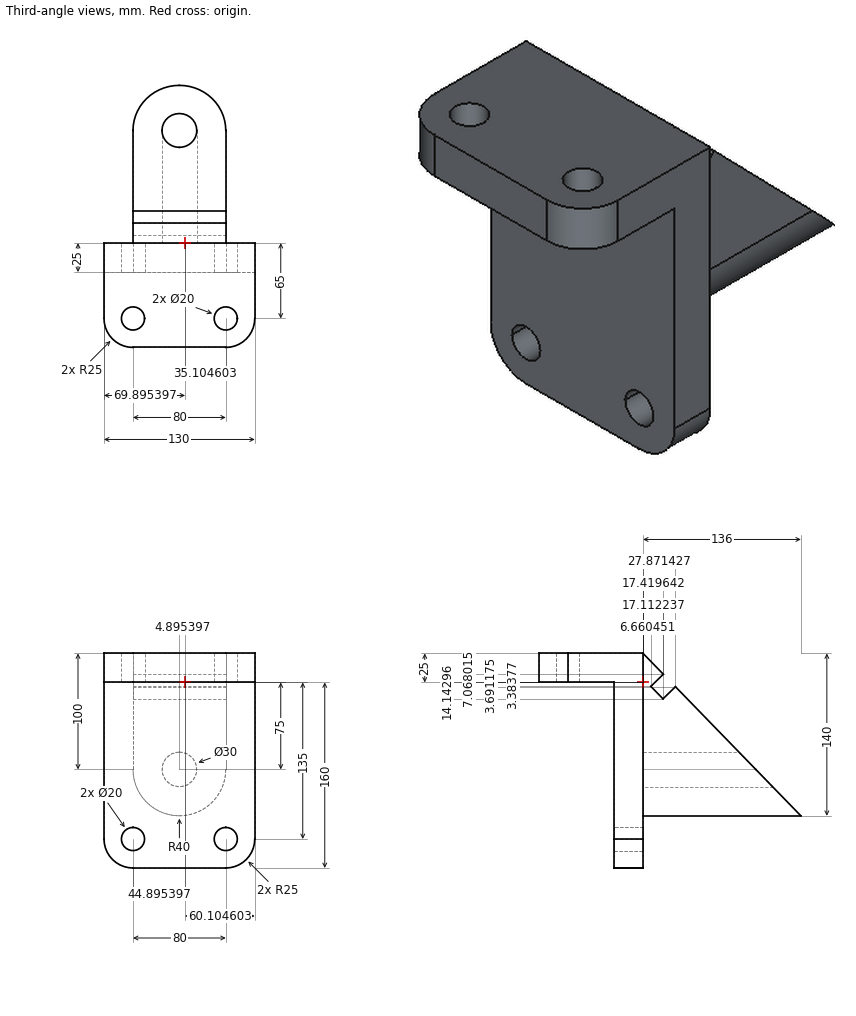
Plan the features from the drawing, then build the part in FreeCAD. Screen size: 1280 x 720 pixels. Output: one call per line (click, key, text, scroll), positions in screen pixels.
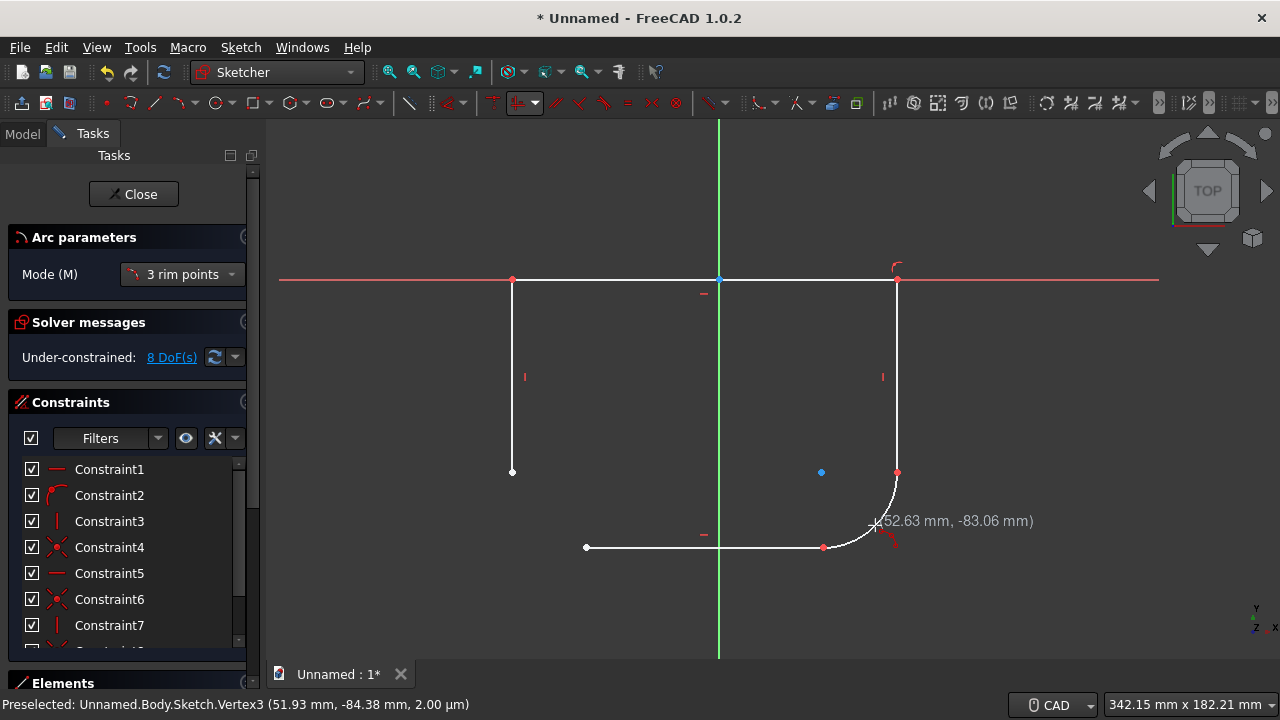
click(512, 473)
click(586, 548)
click(534, 525)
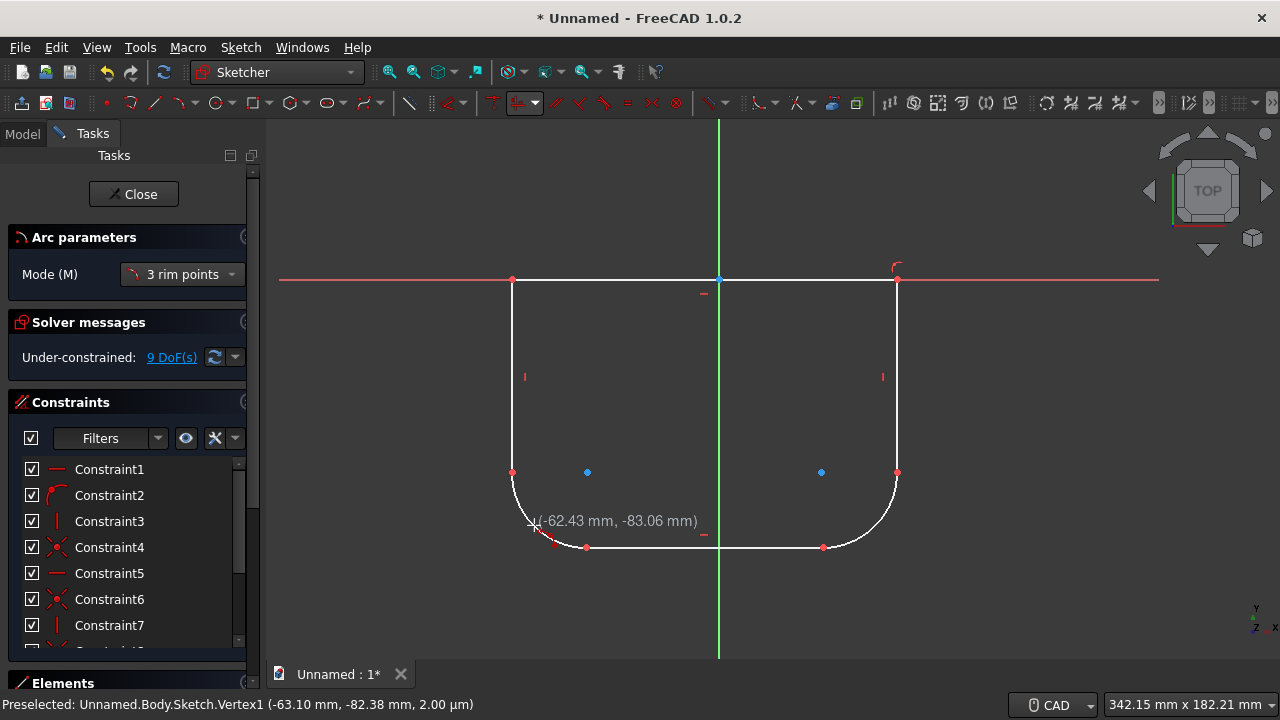
click(216, 104)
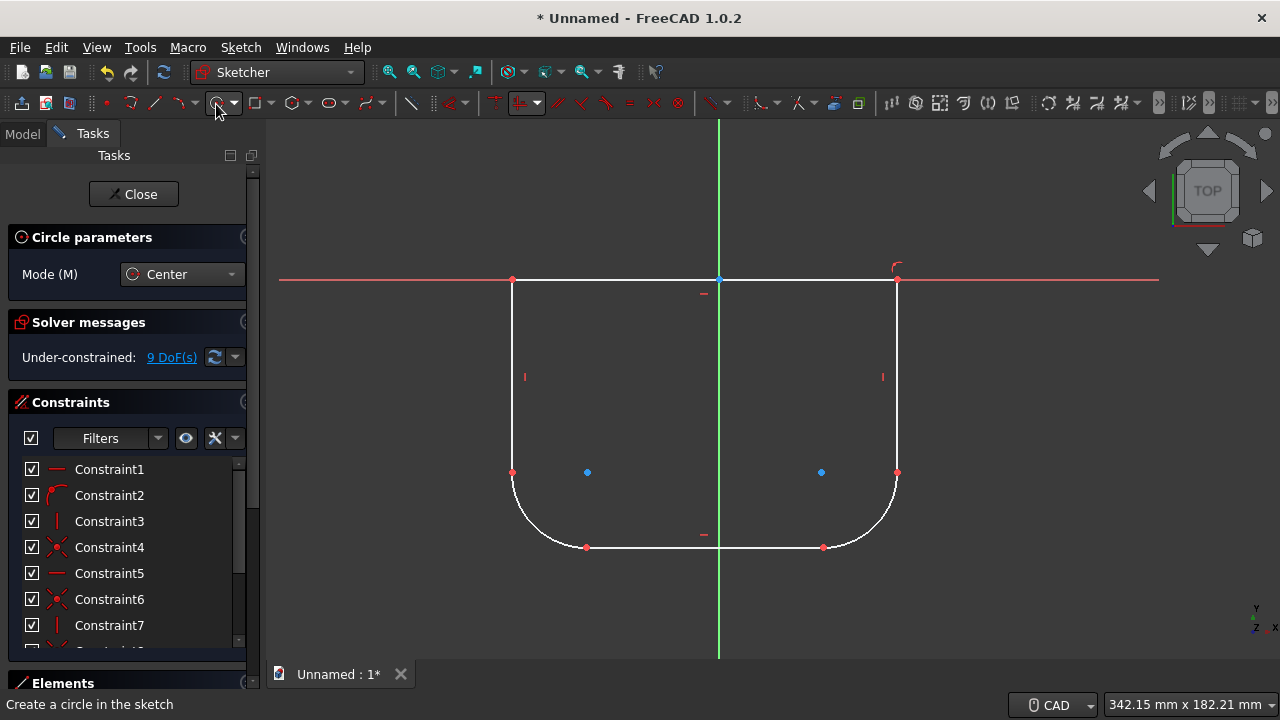
click(823, 472)
click(844, 452)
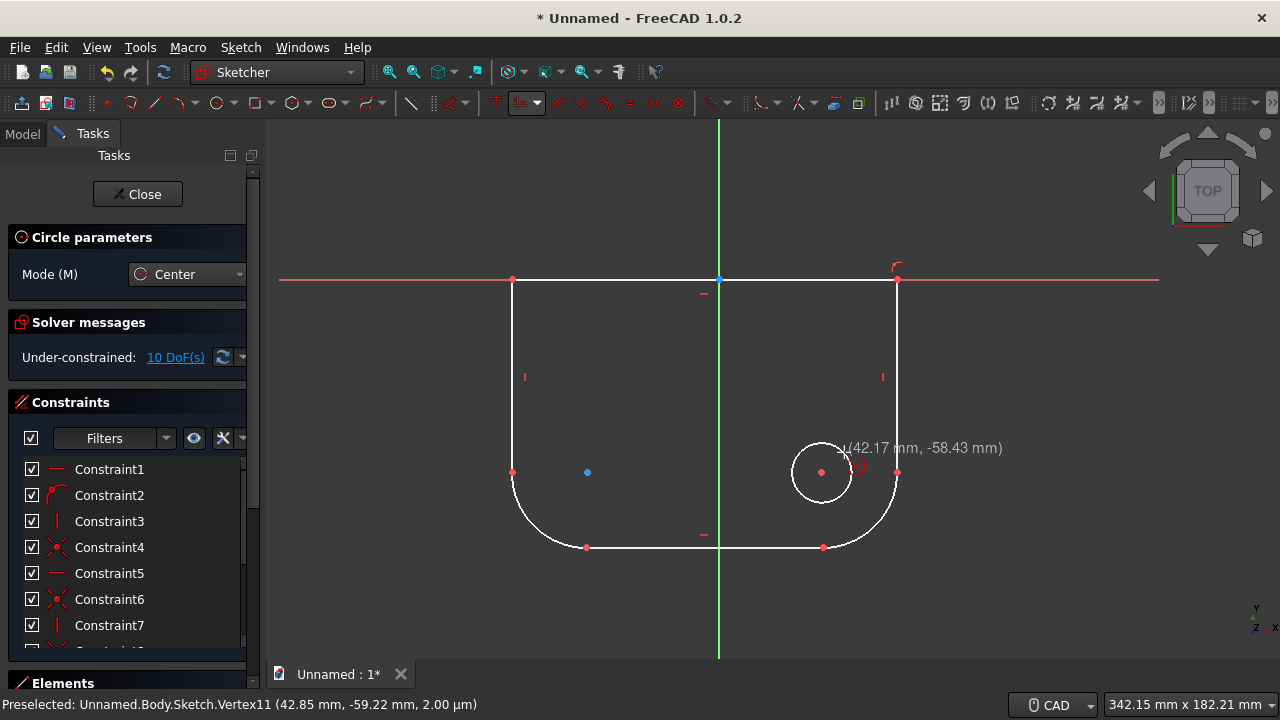
click(586, 472)
click(607, 452)
key(Escape)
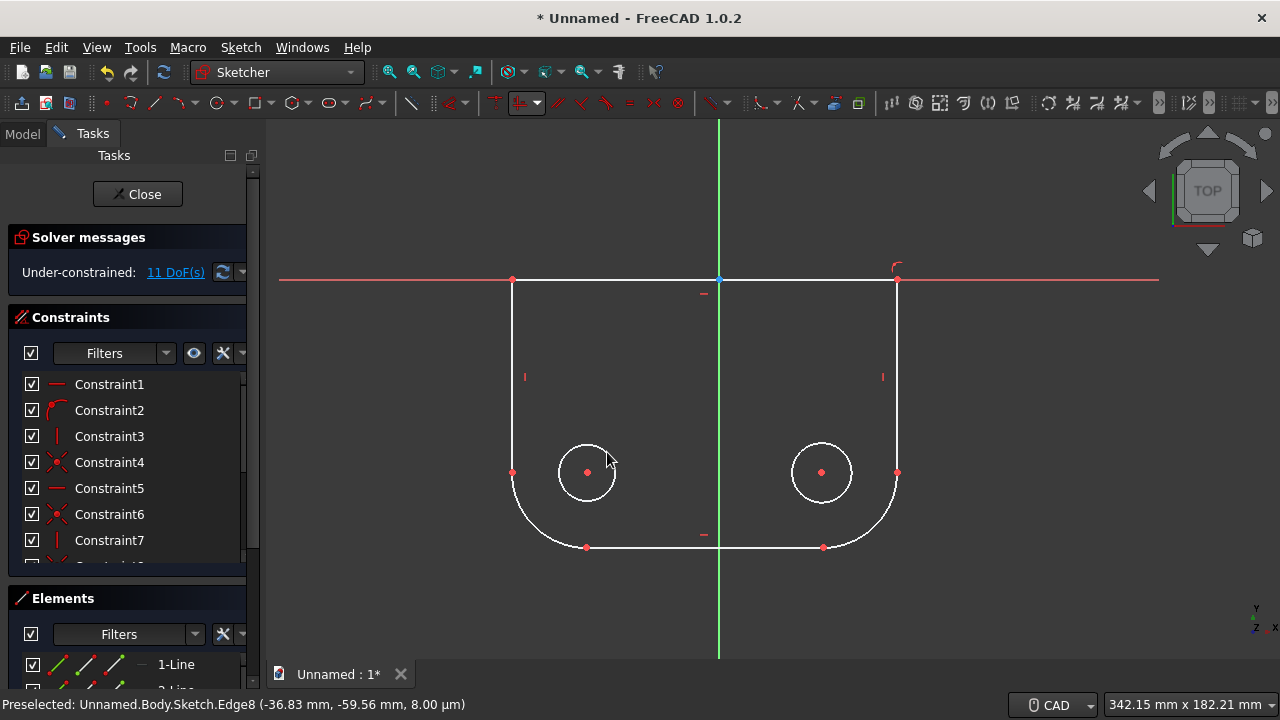
click(657, 548)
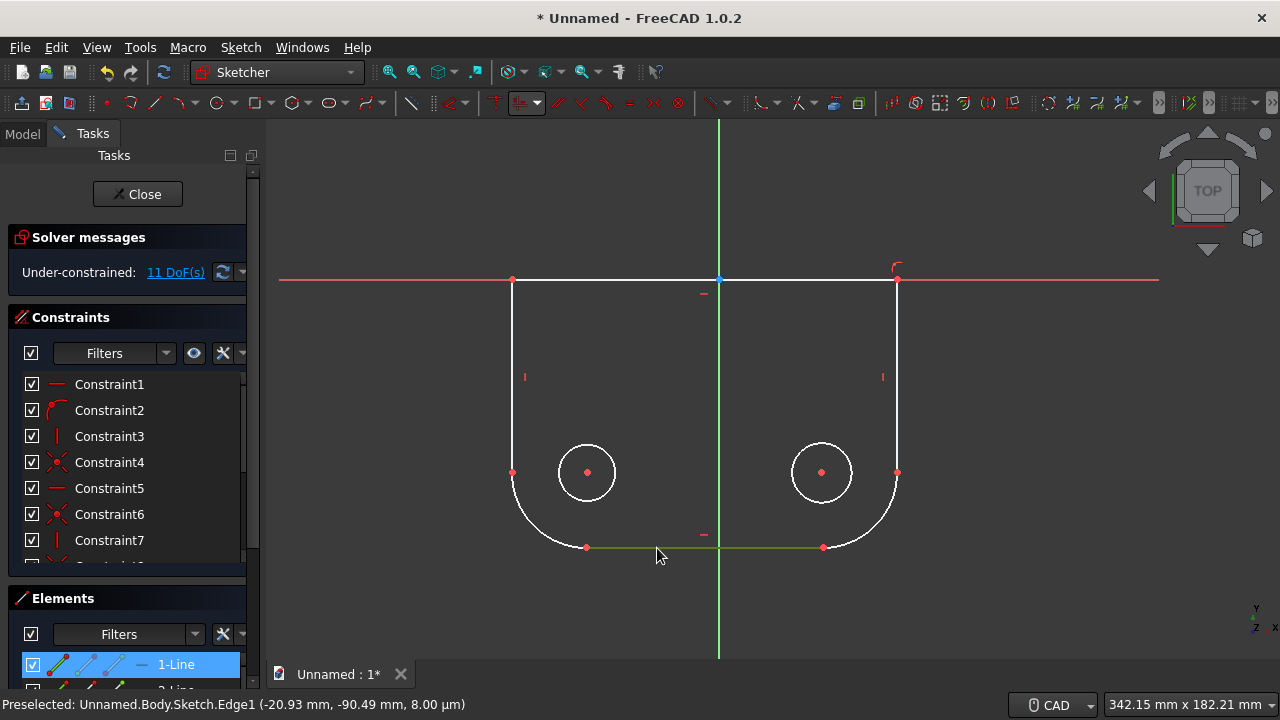
click(857, 539)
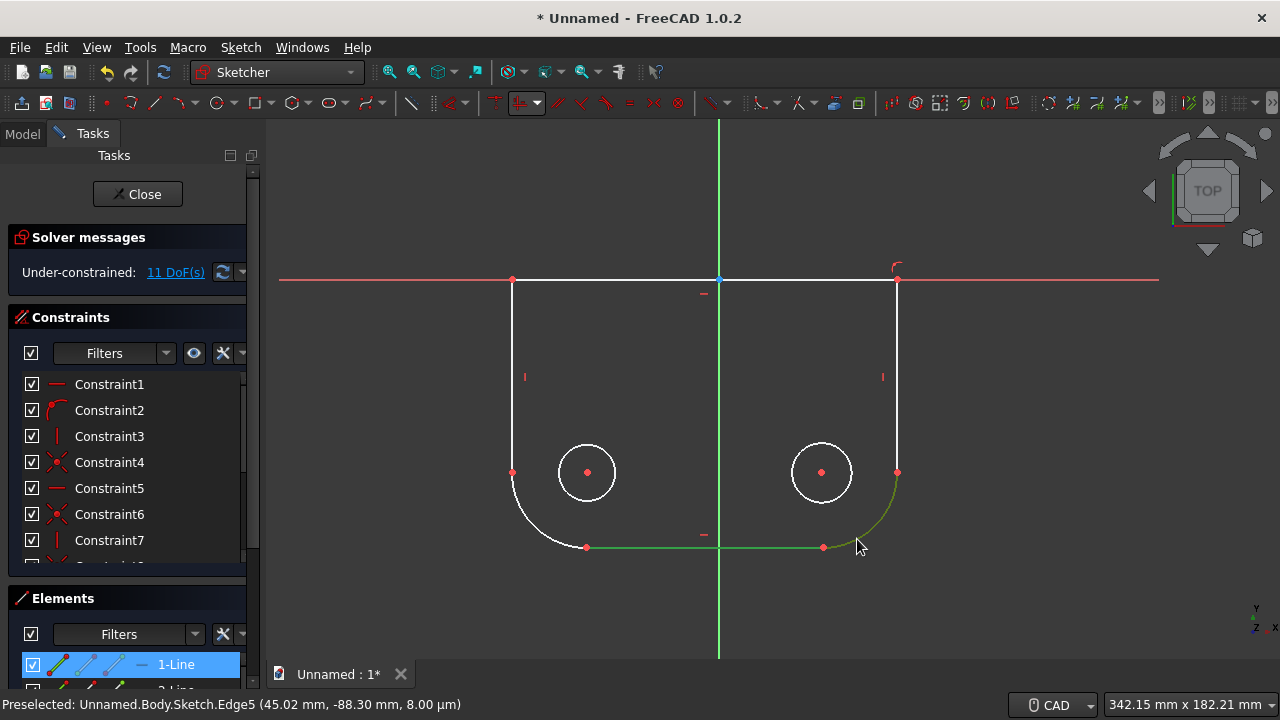
key(t)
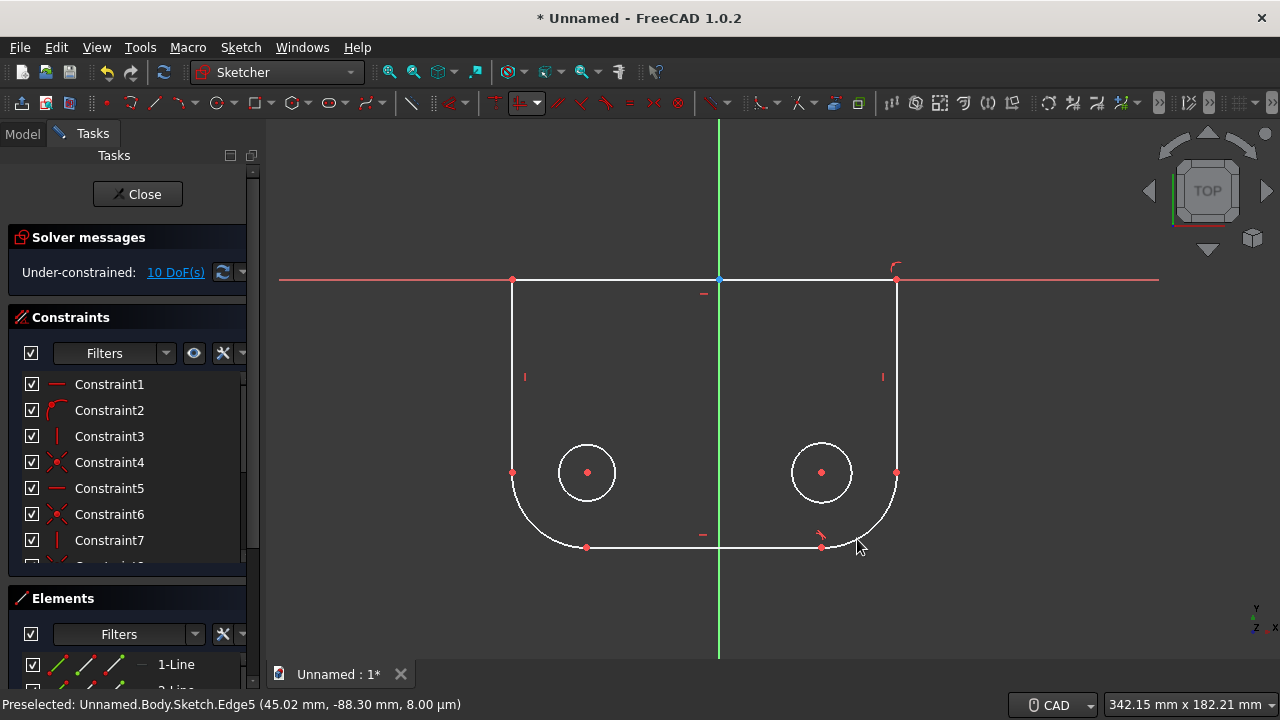
click(657, 548)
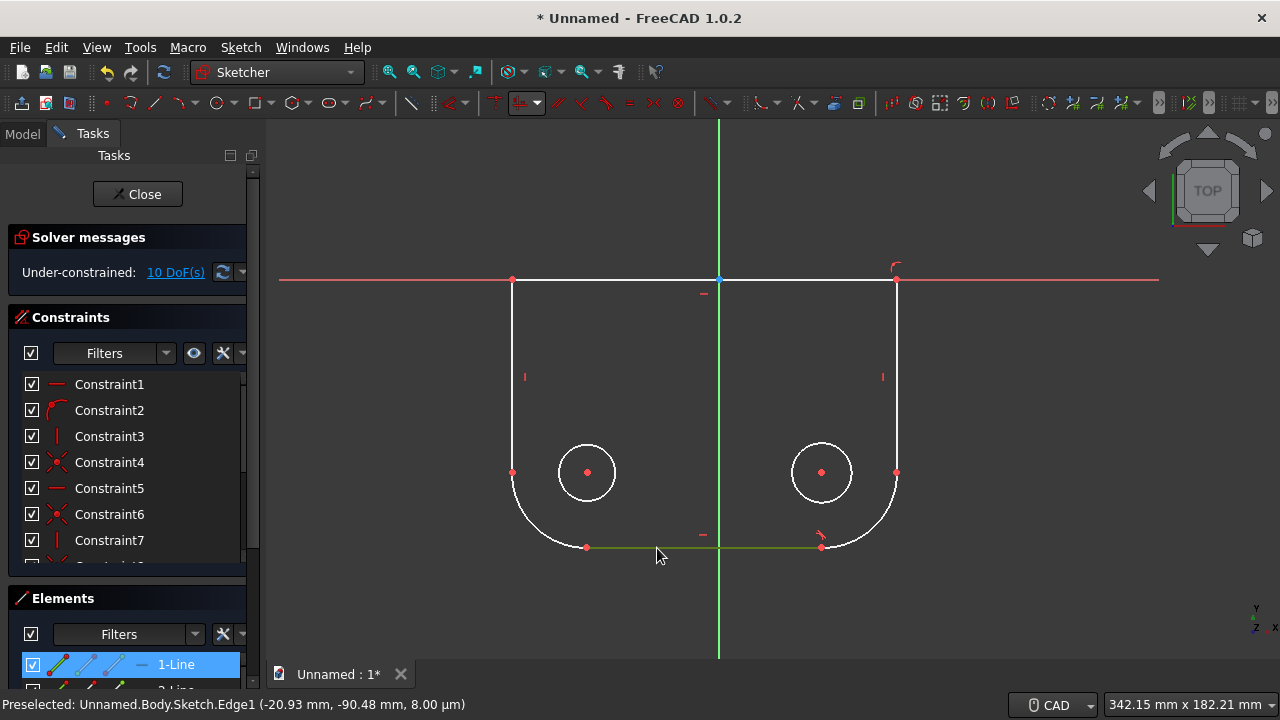
click(520, 507)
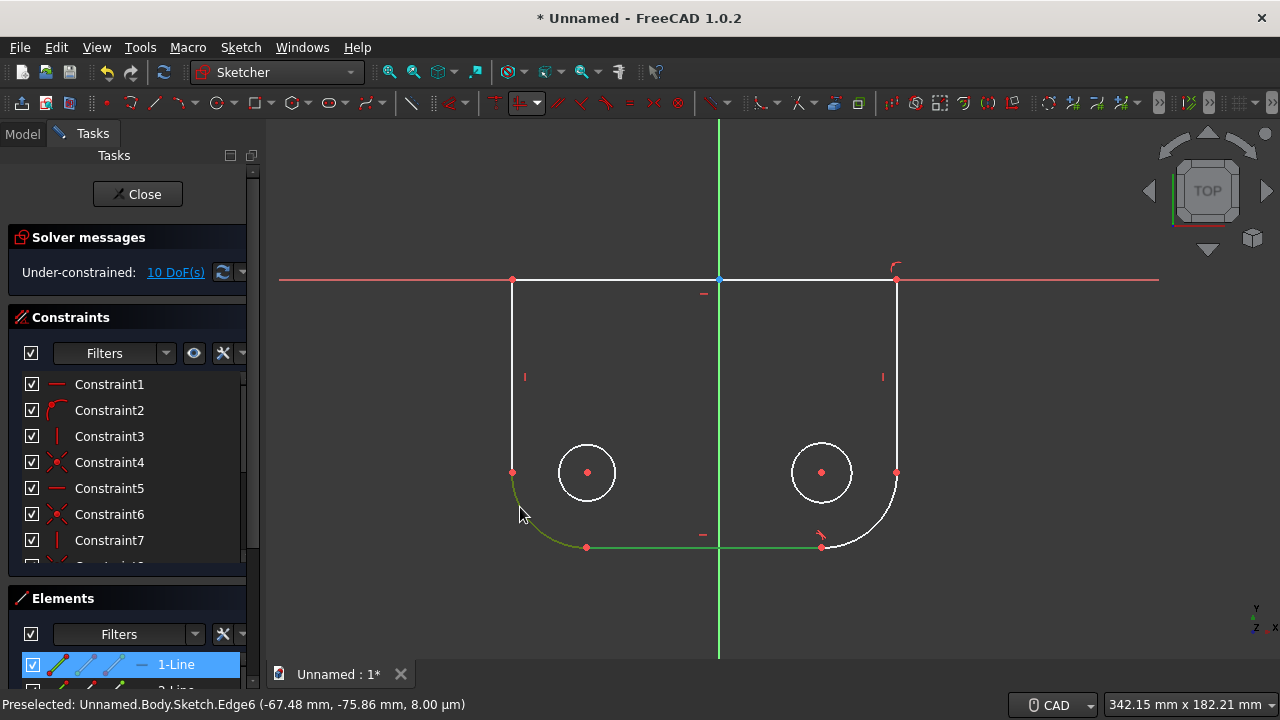
click(606, 104)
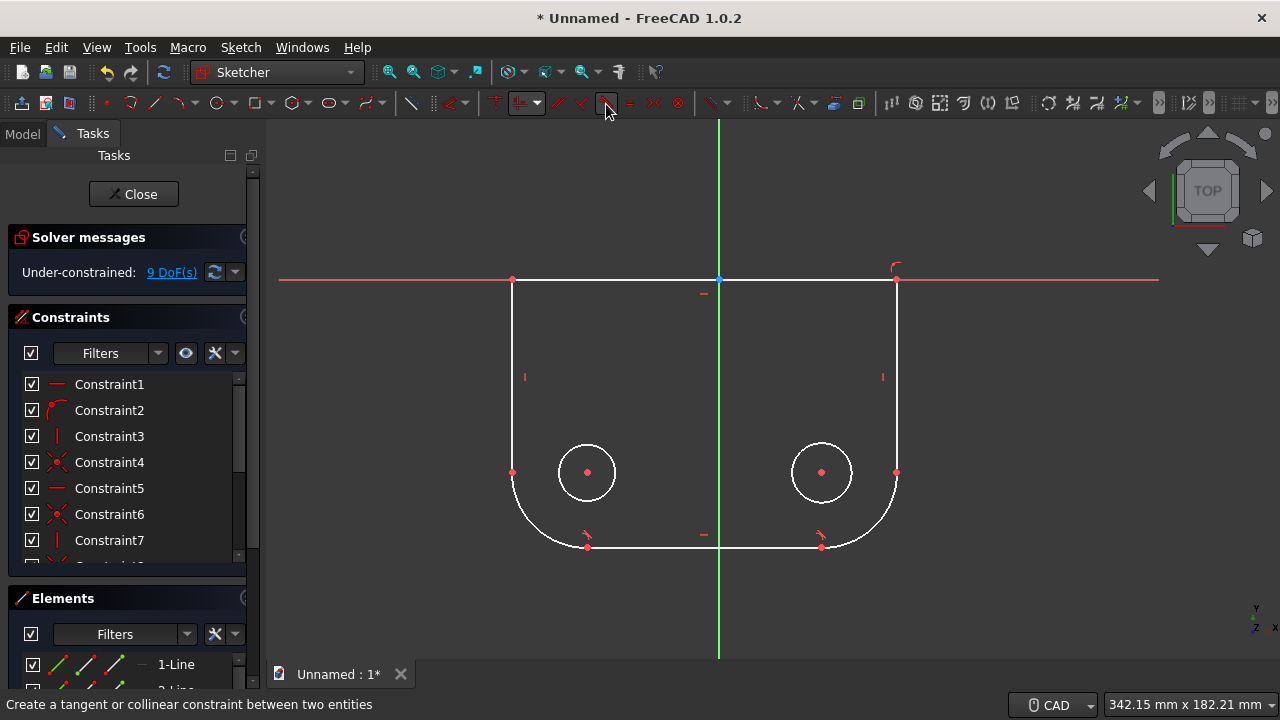
click(897, 415)